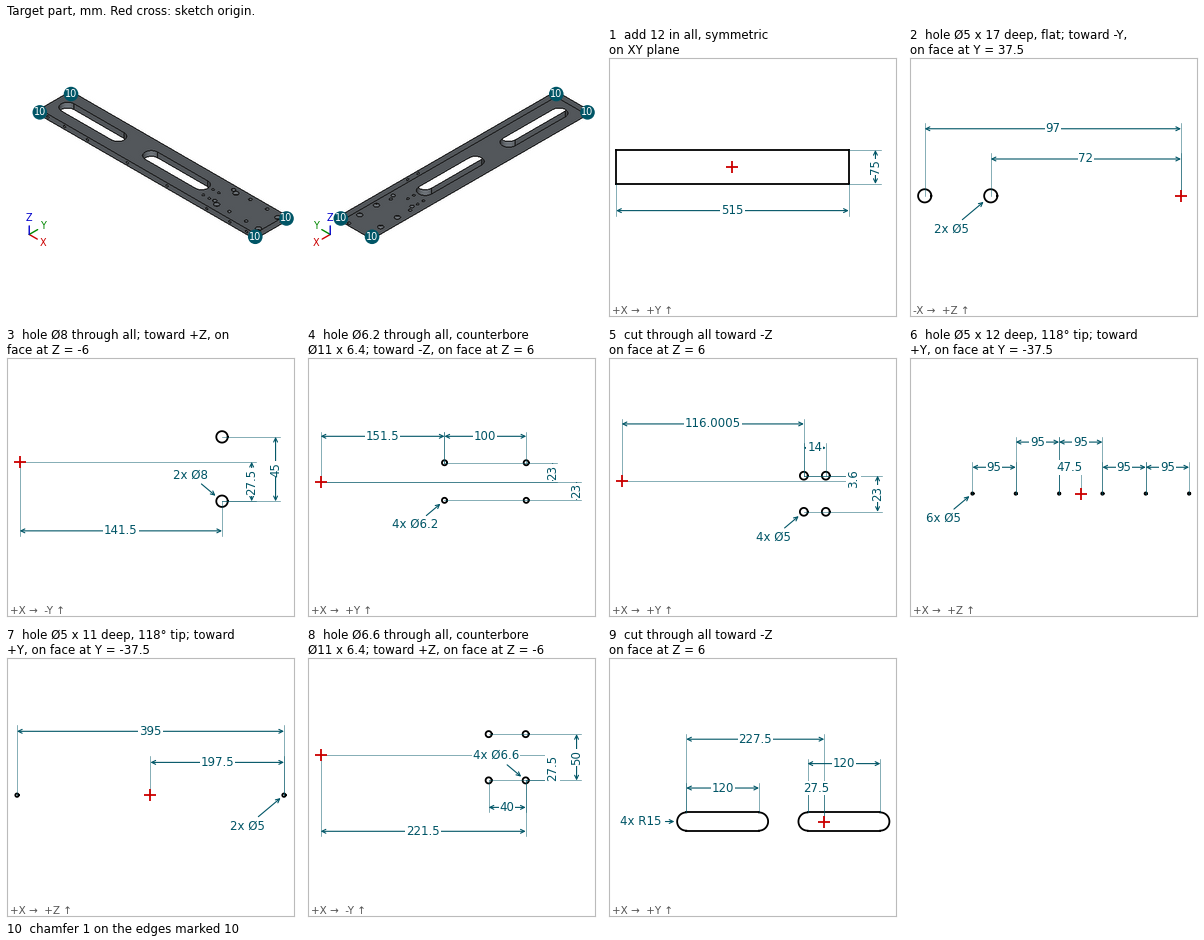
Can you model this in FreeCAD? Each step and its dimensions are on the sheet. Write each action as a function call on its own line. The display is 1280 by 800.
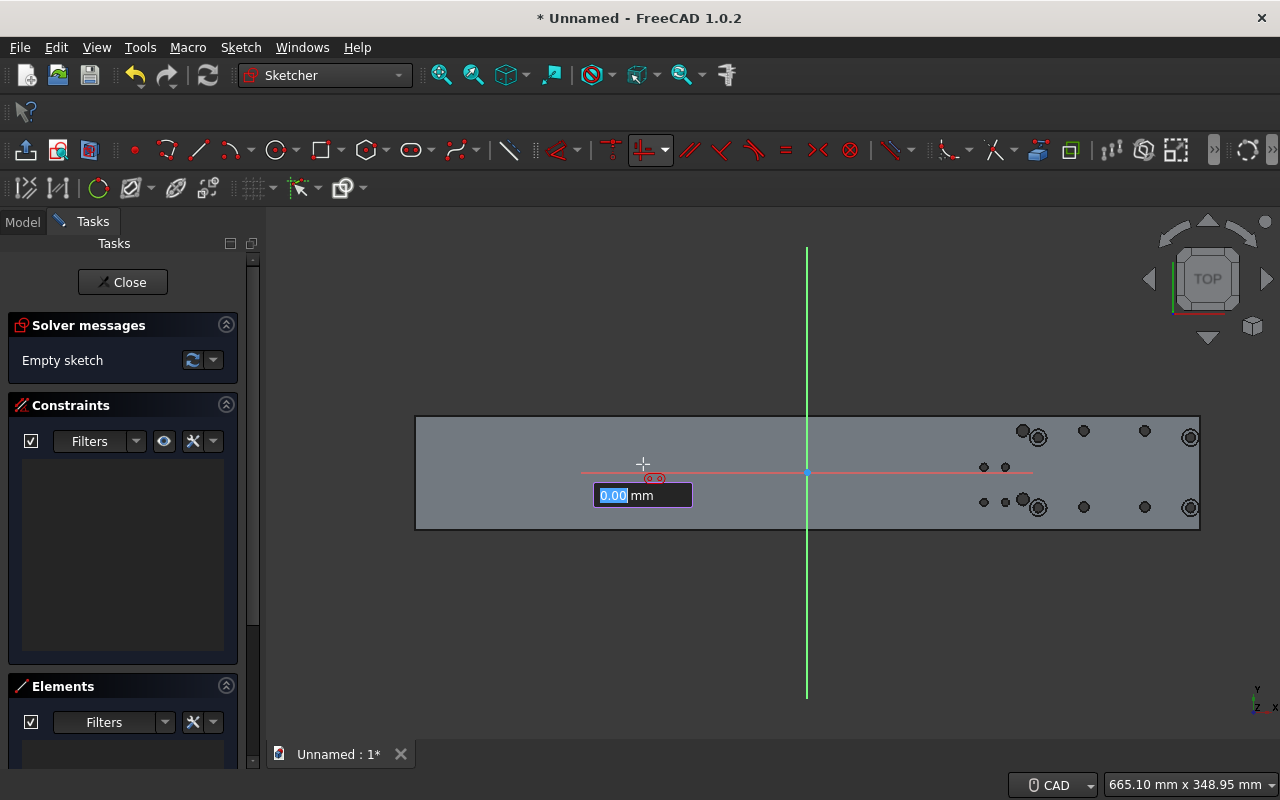
click(552, 450)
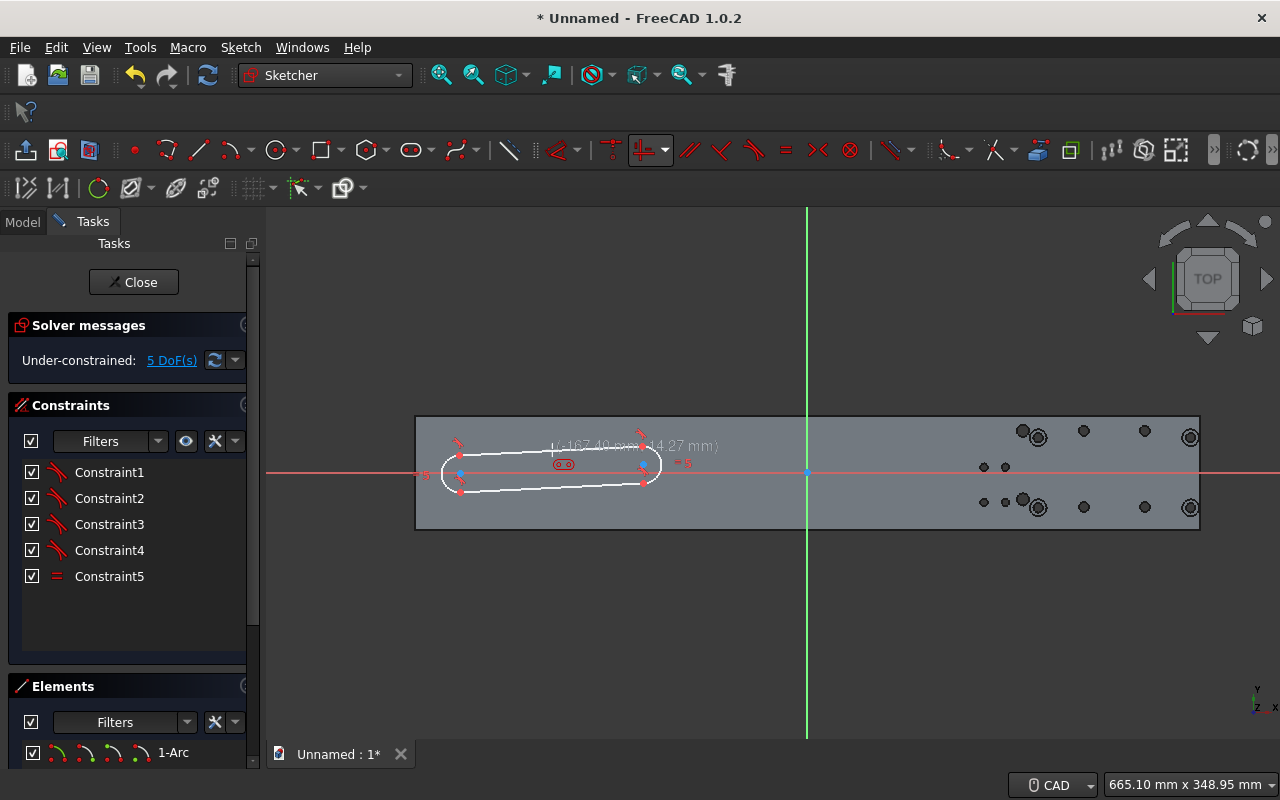
click(765, 473)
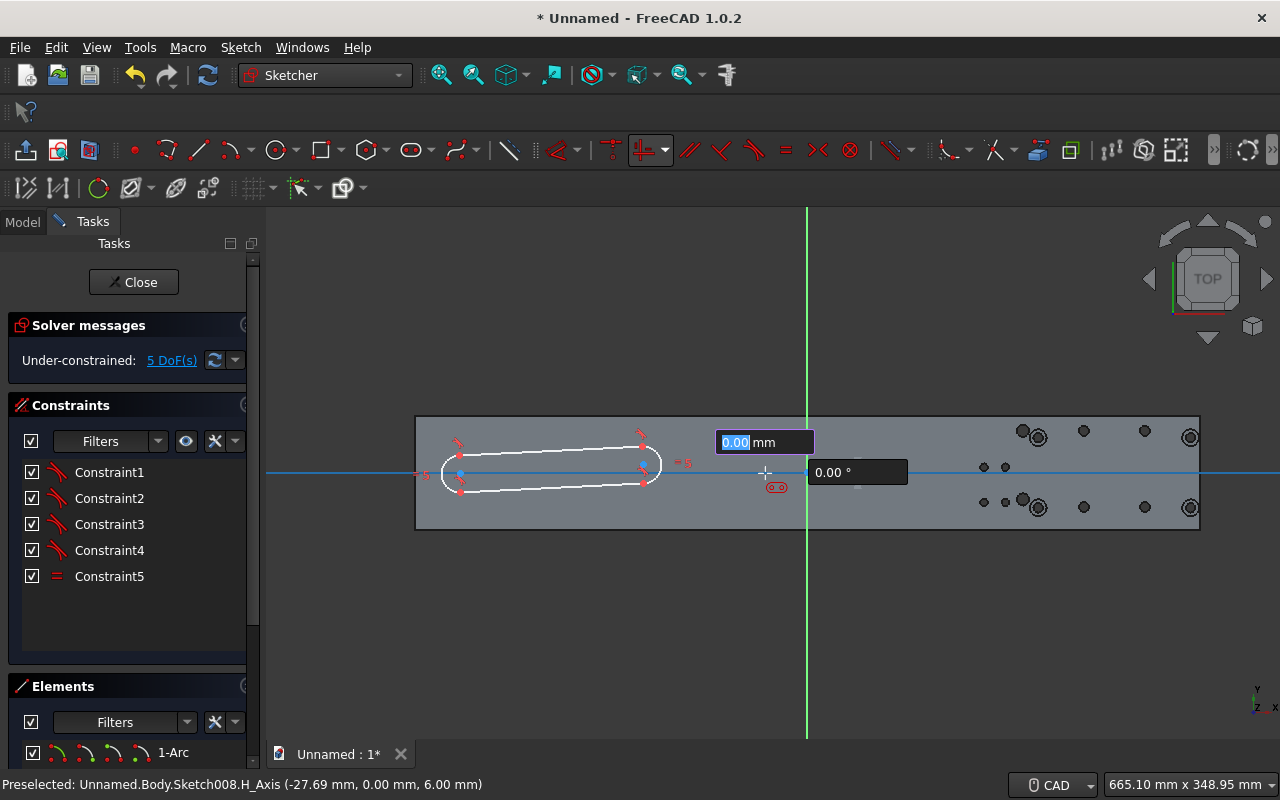
click(948, 464)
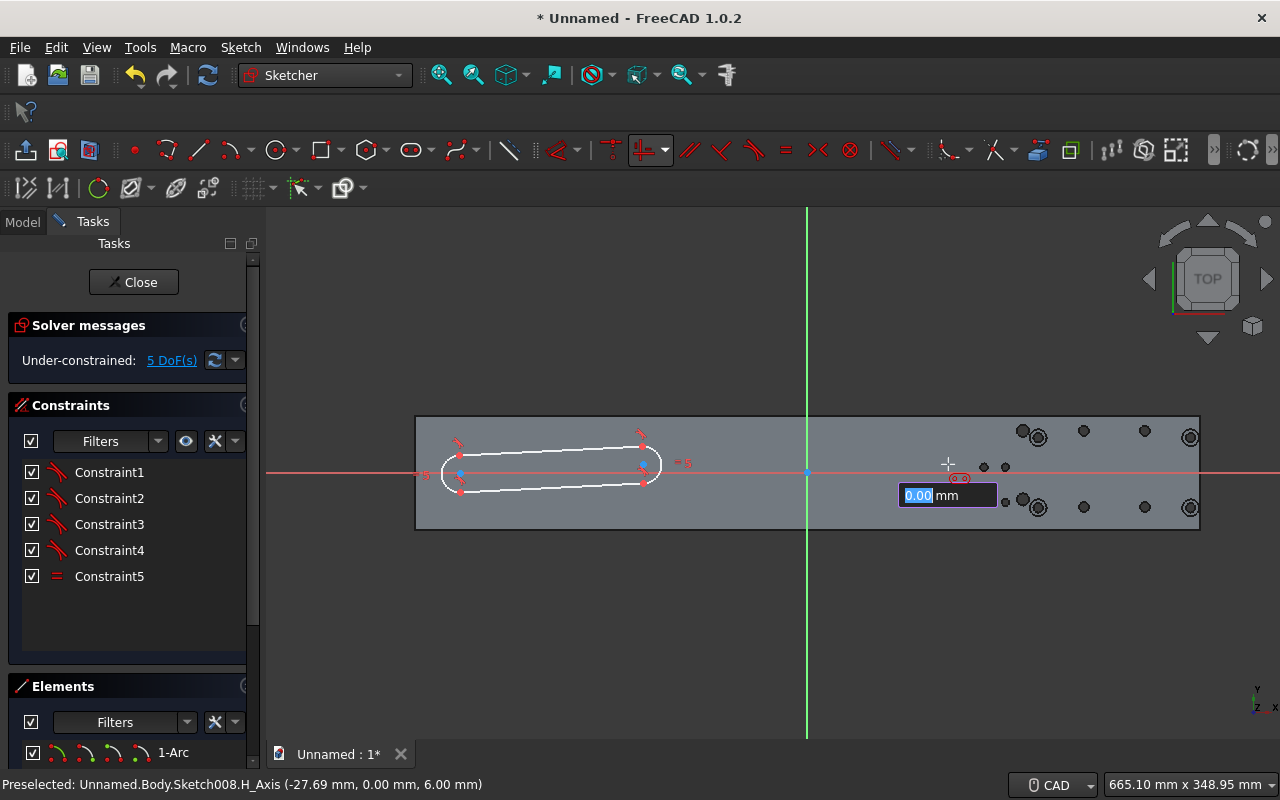
click(857, 450)
key(Escape)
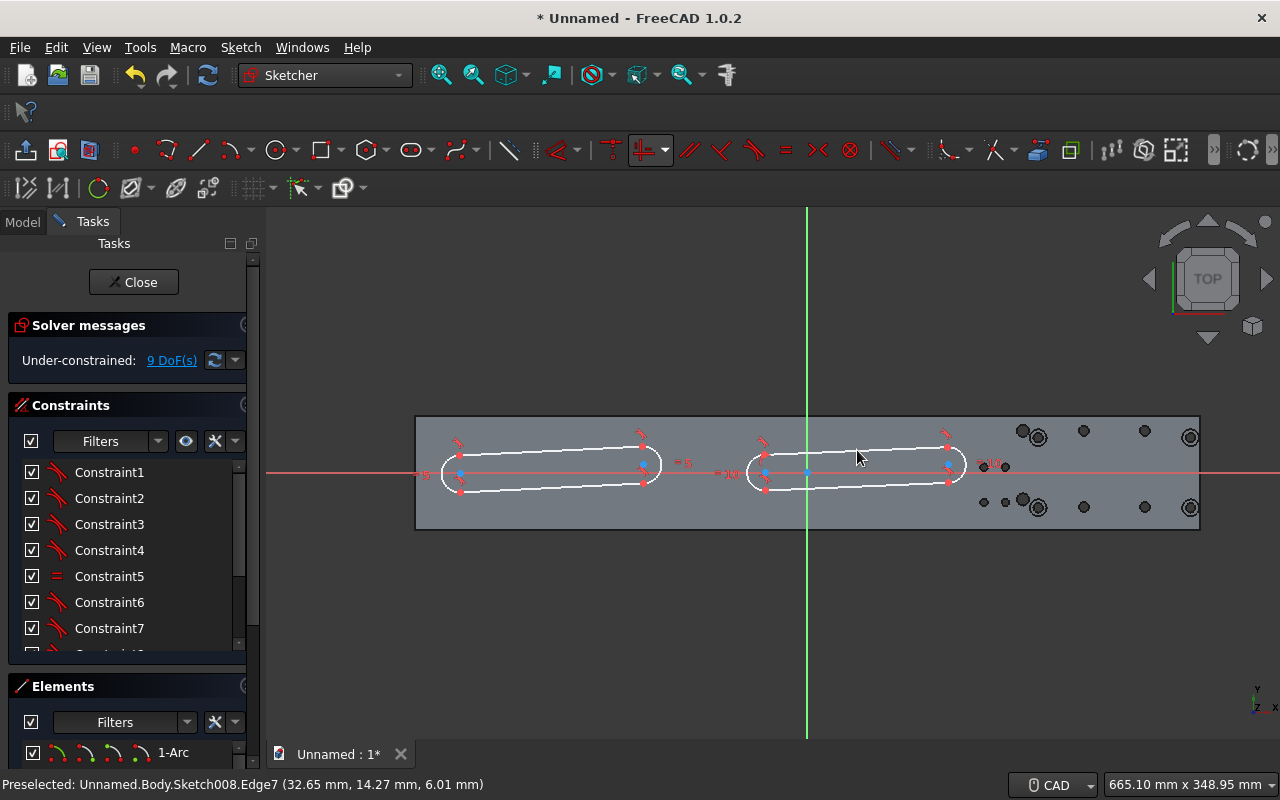
click(514, 453)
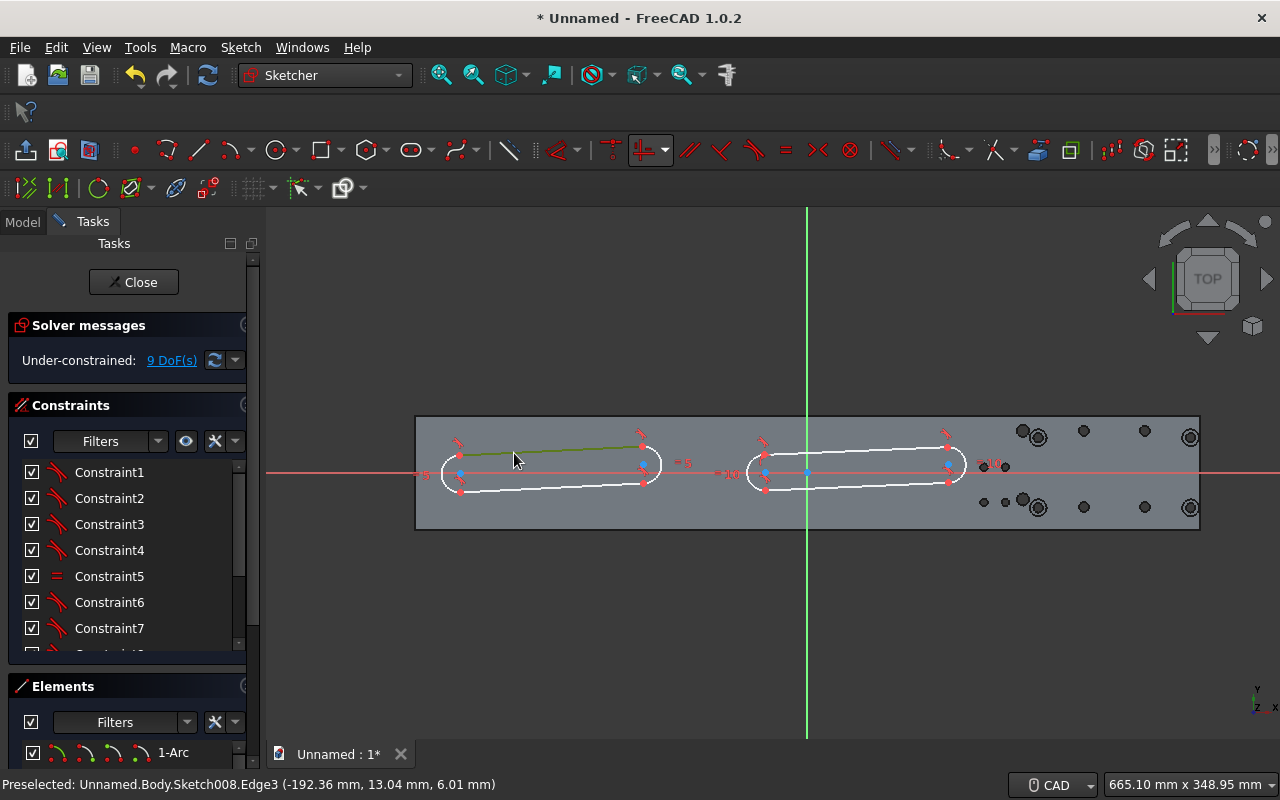
key(h)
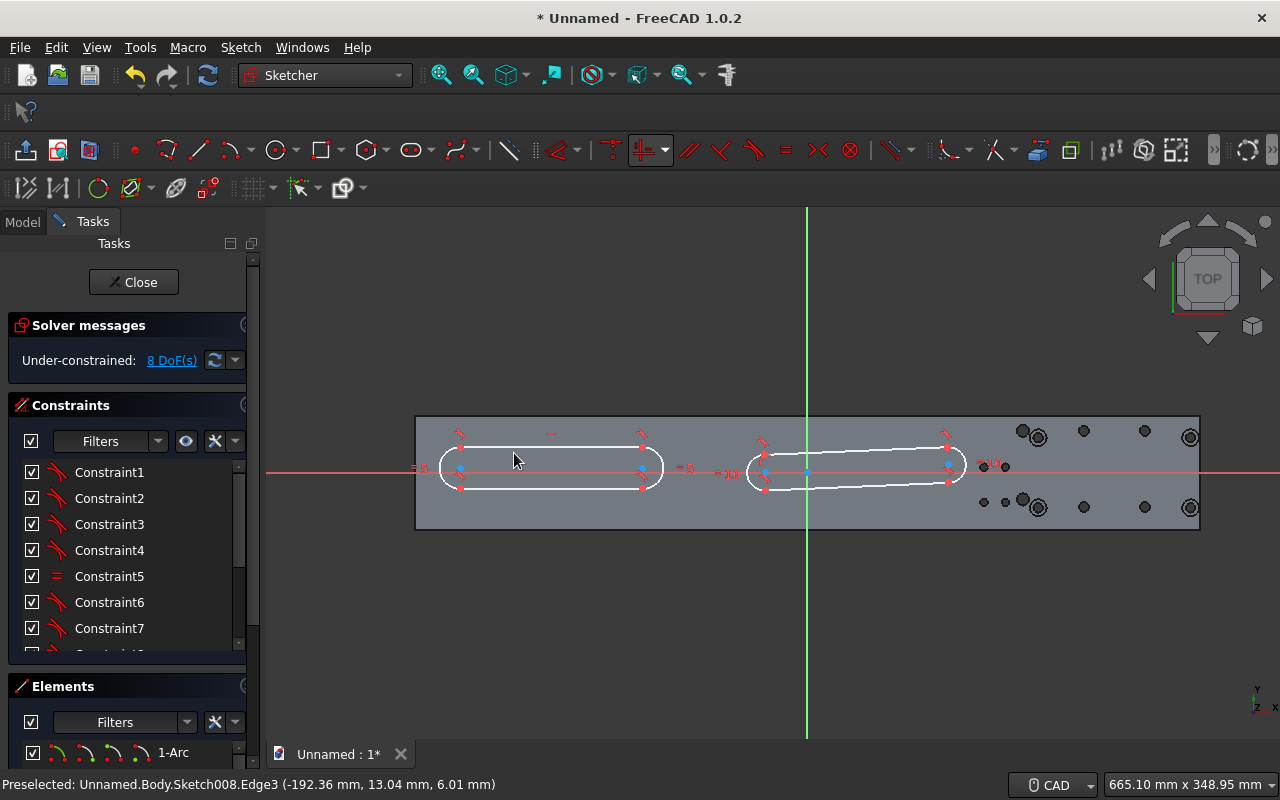
click(819, 453)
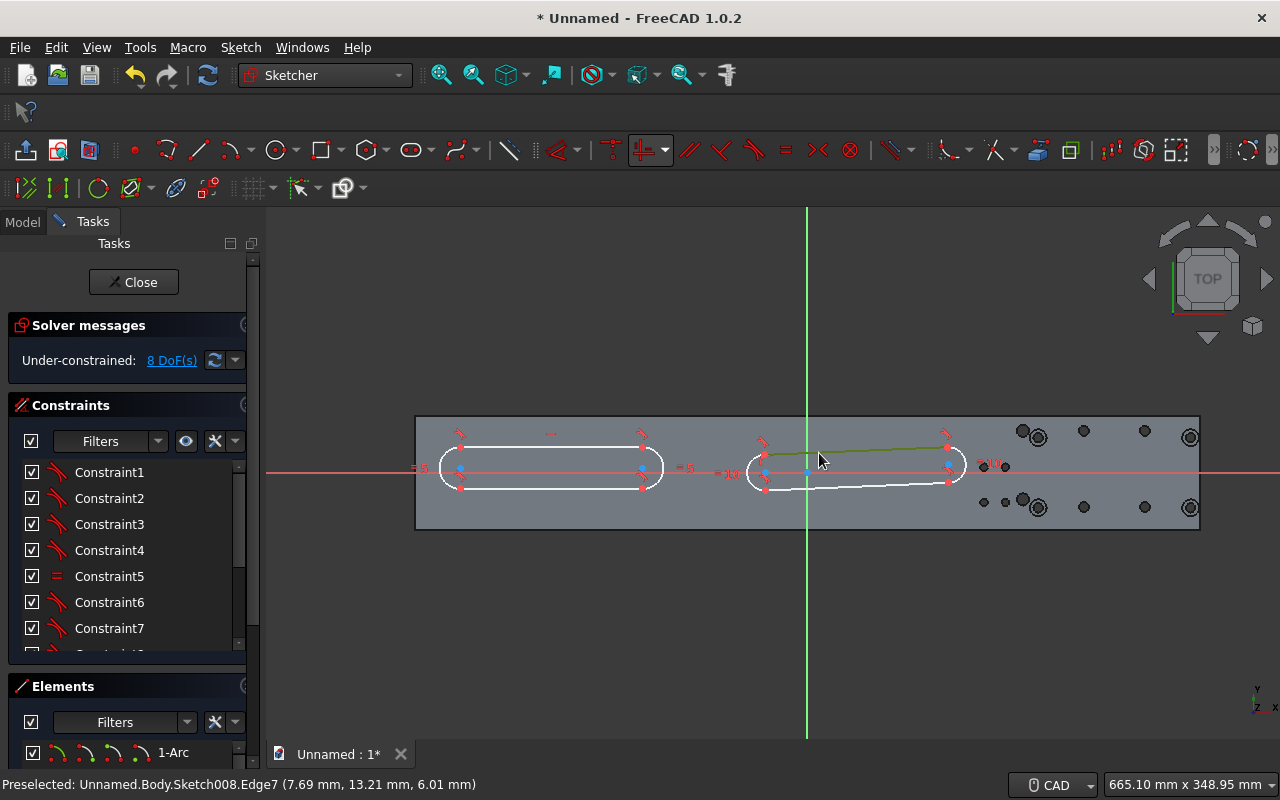
click(668, 150)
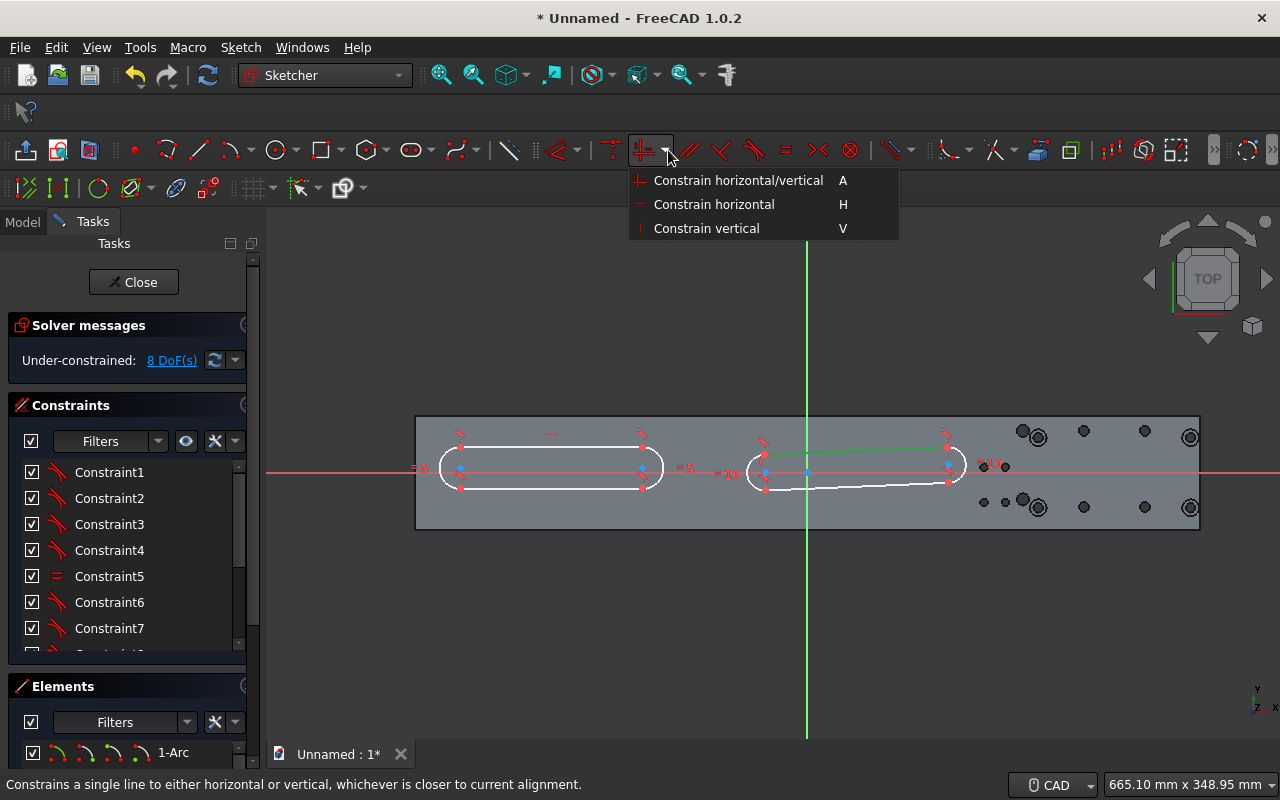
click(764, 204)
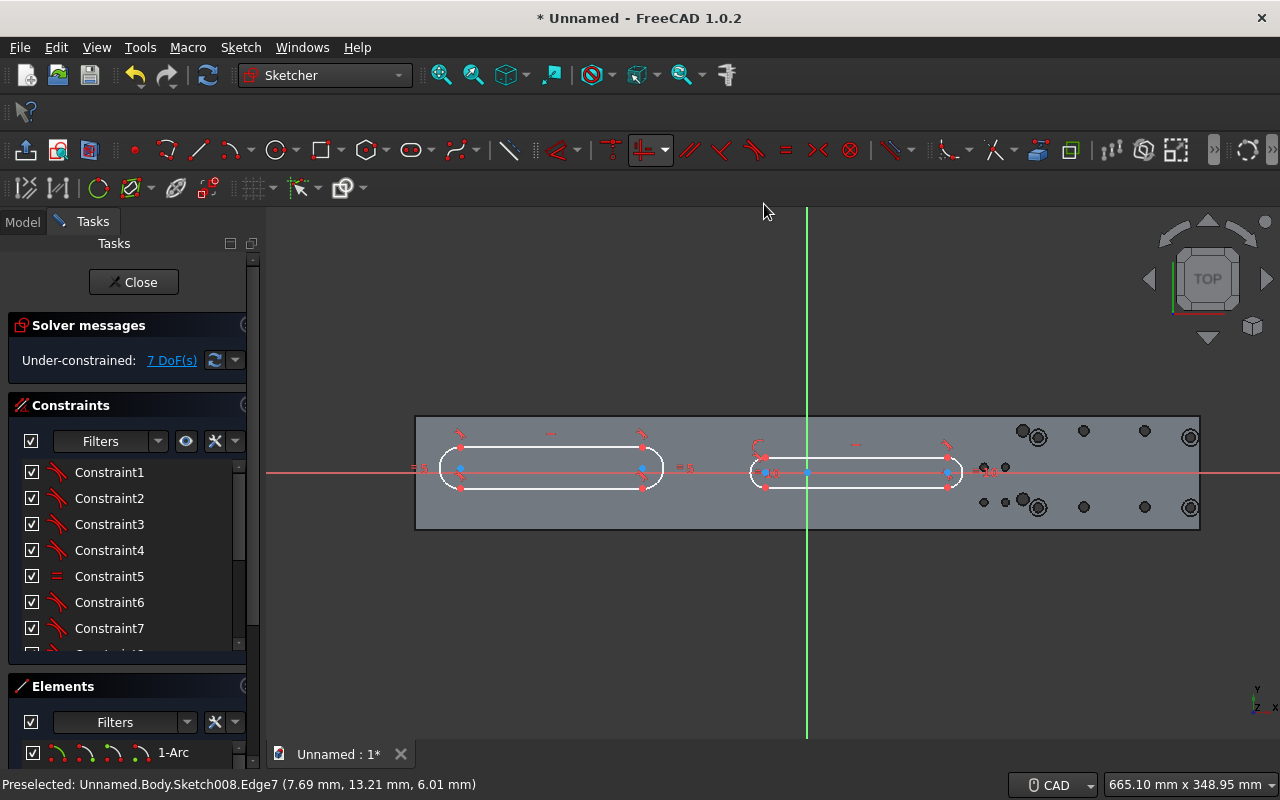
click(444, 456)